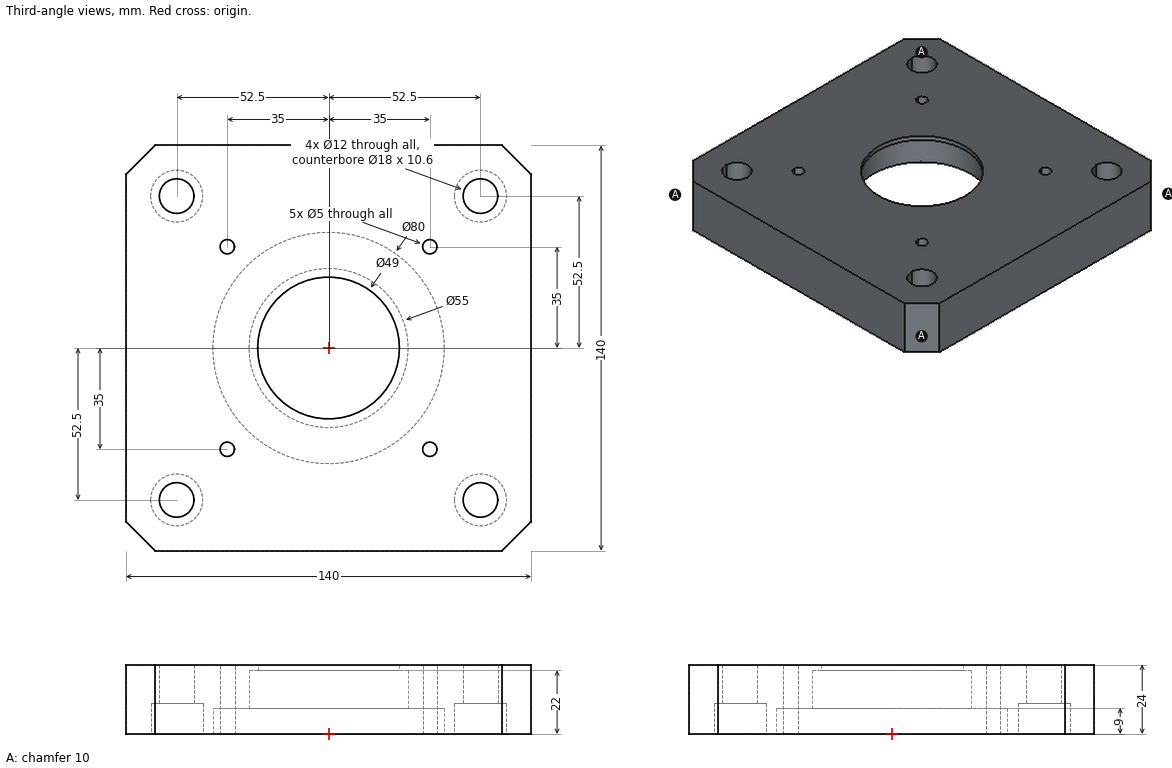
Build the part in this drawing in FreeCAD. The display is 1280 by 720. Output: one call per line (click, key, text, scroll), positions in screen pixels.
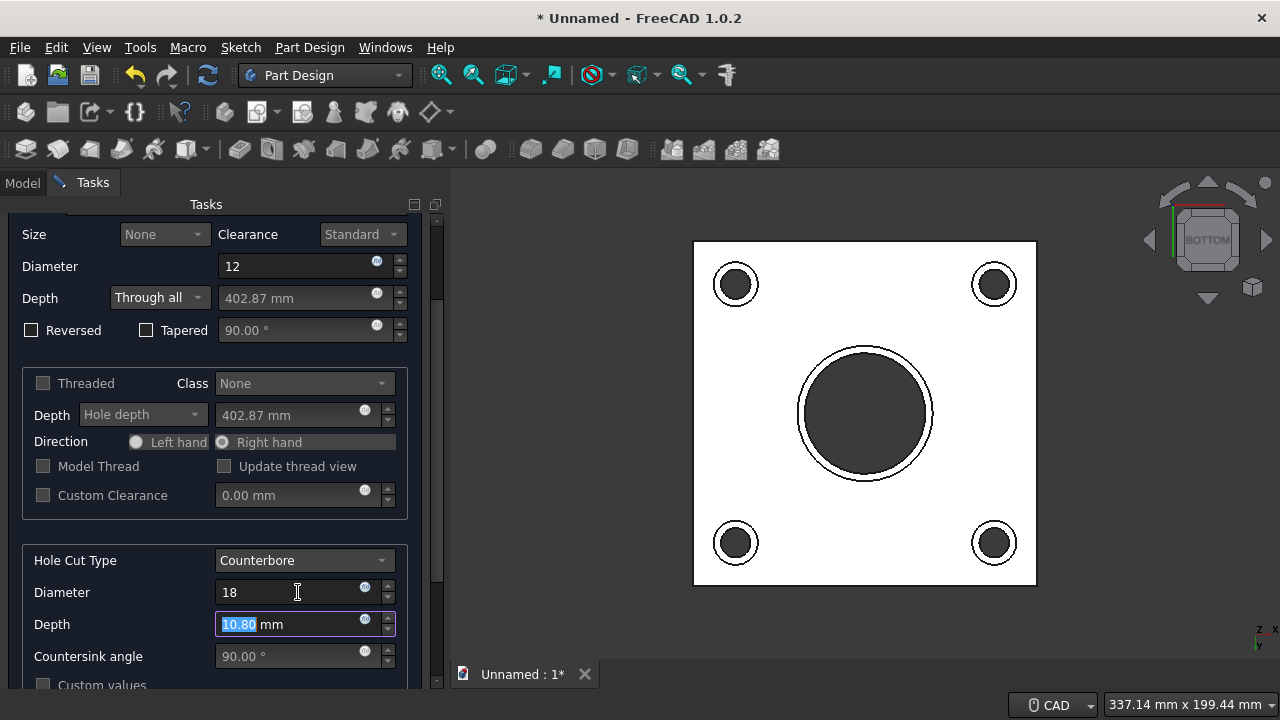
text(10.6)
key(Tab)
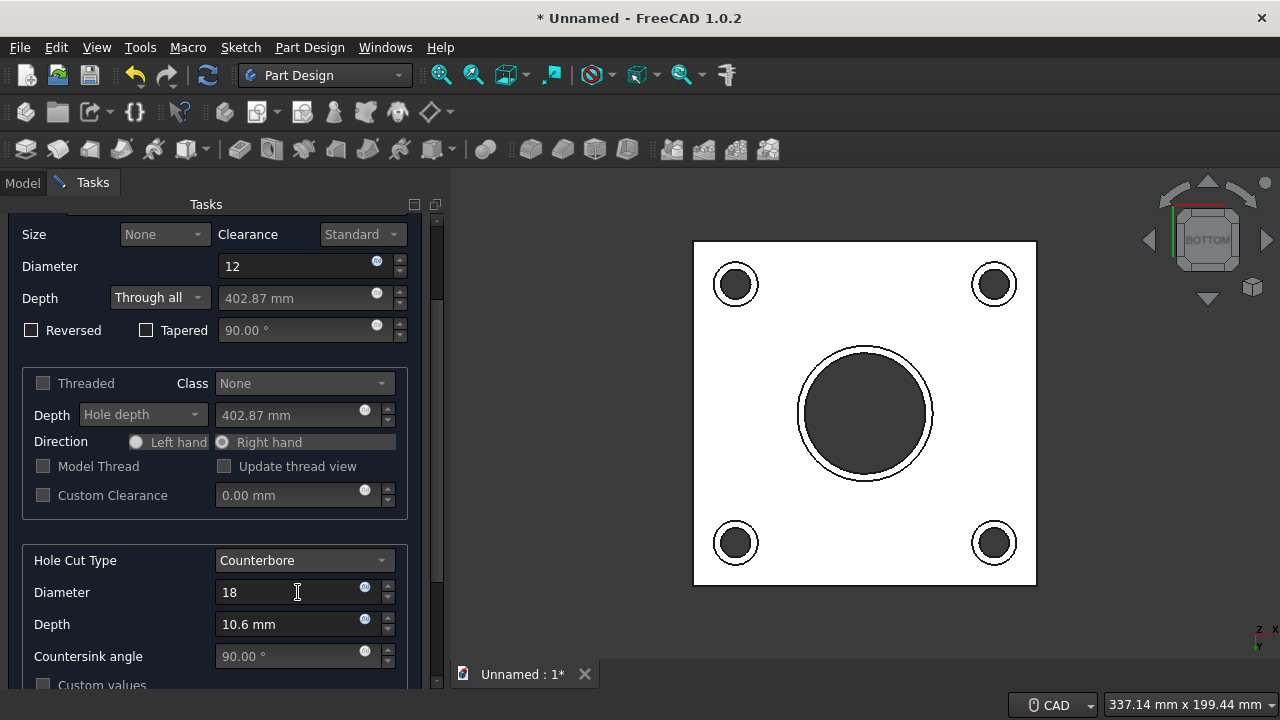
scroll(437, 451, up, 3)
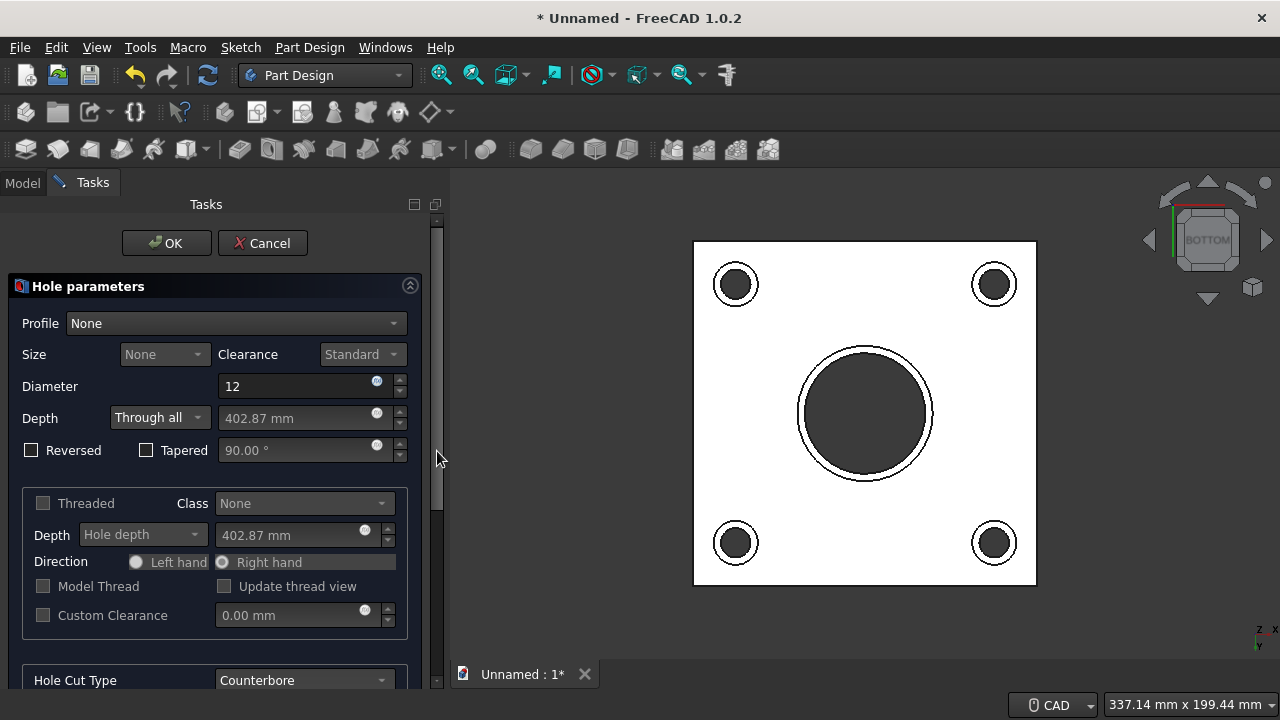
click(167, 243)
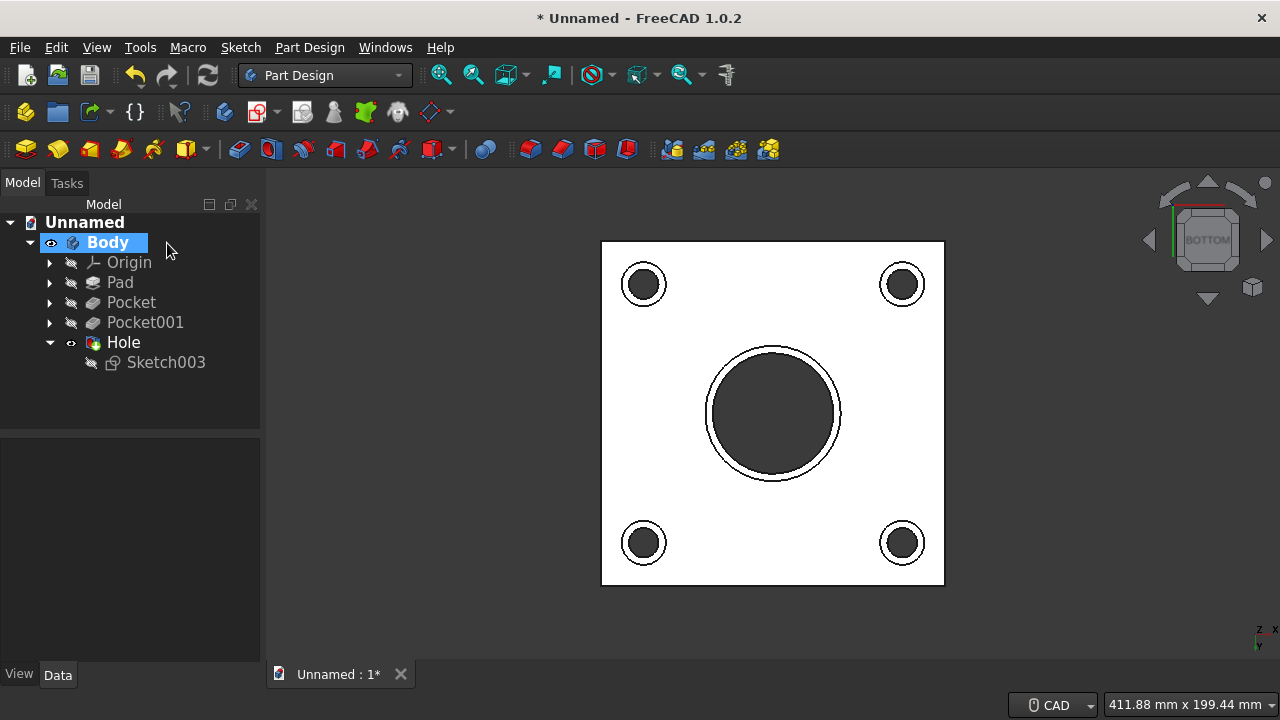
key(0)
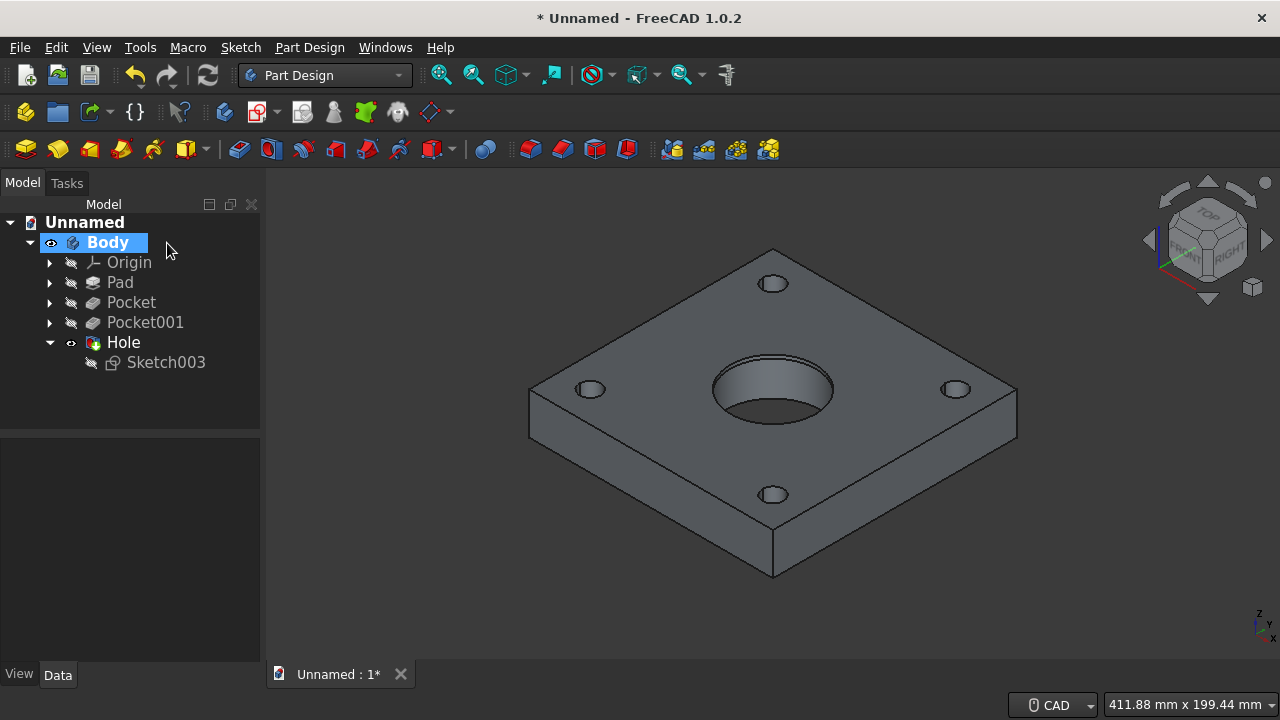
click(773, 553)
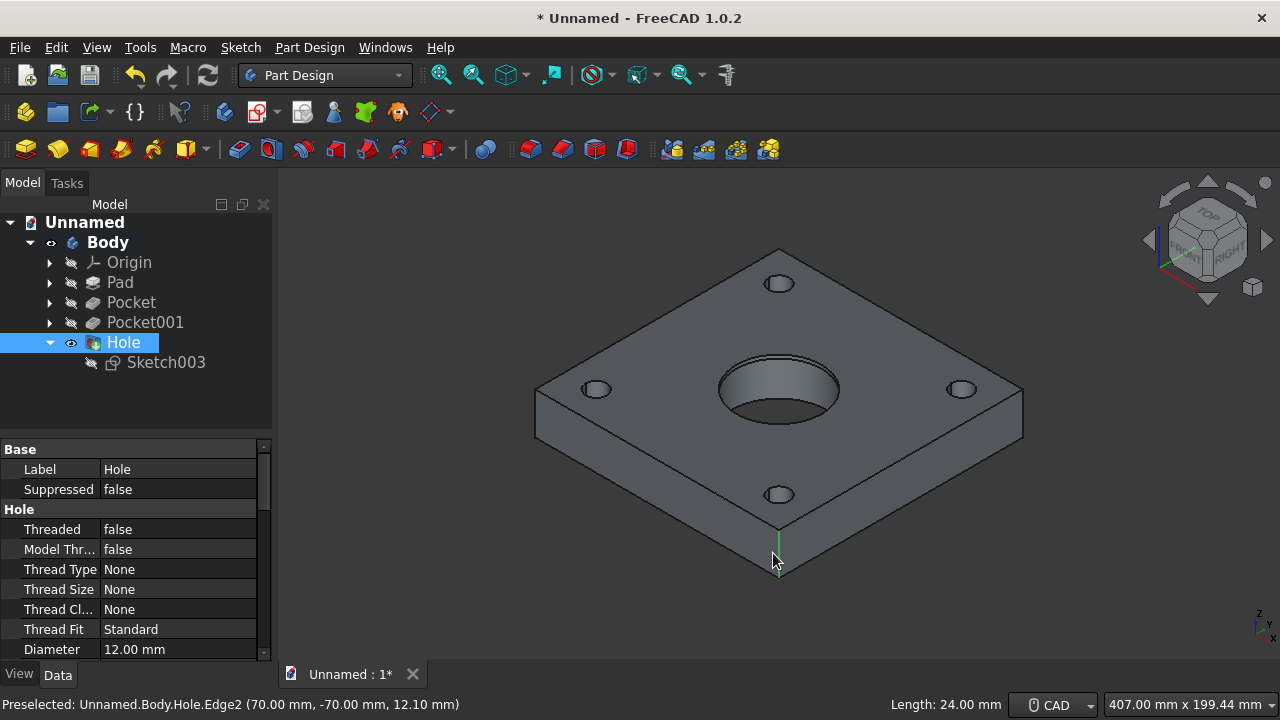
key(2)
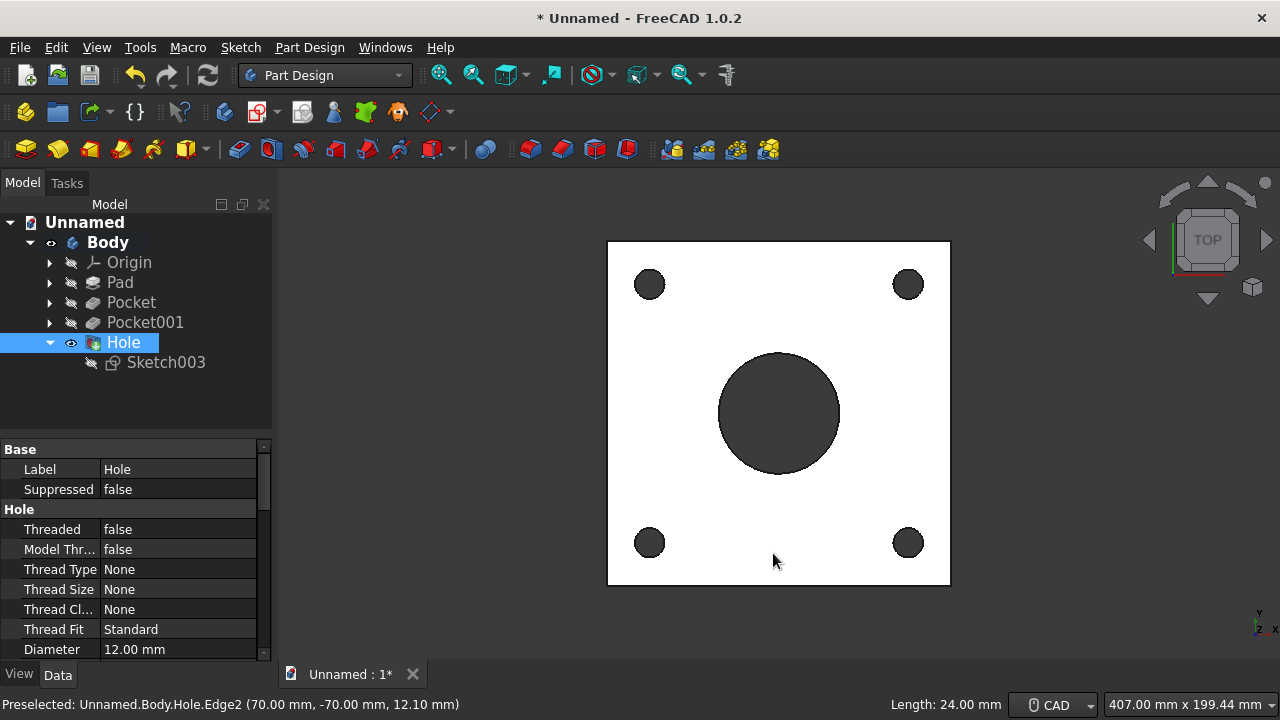
key(1)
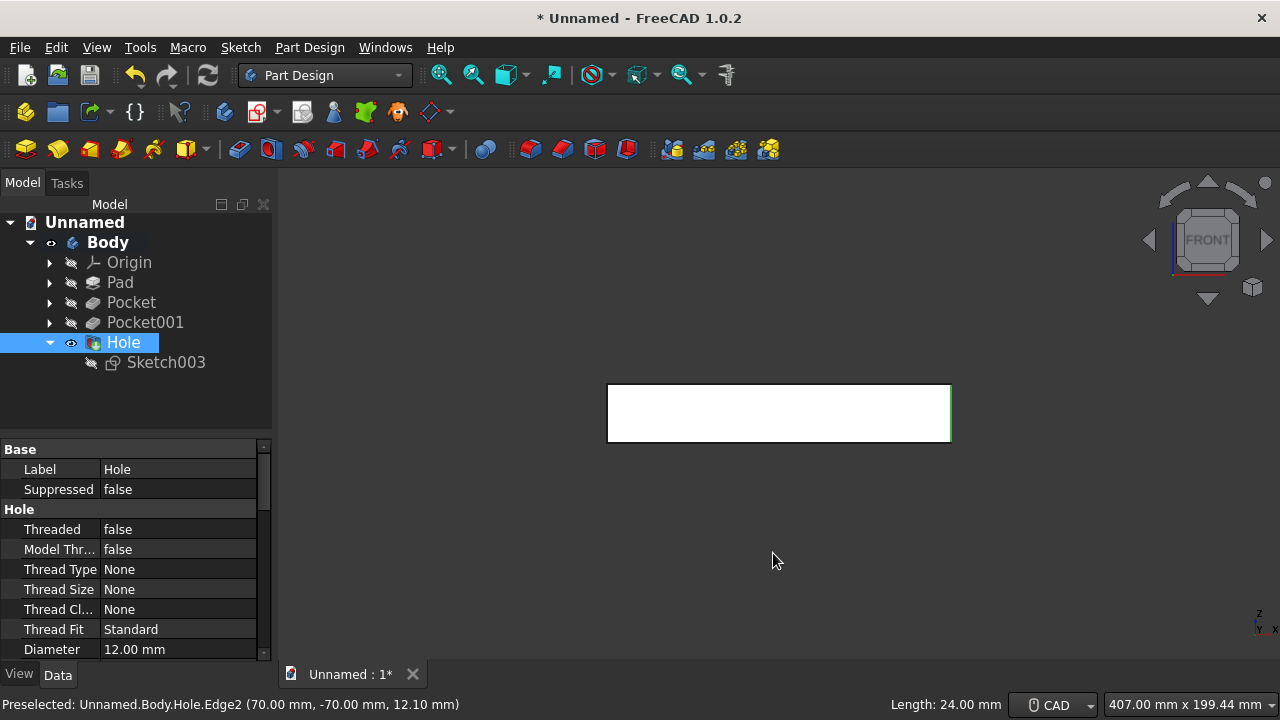
click(442, 76)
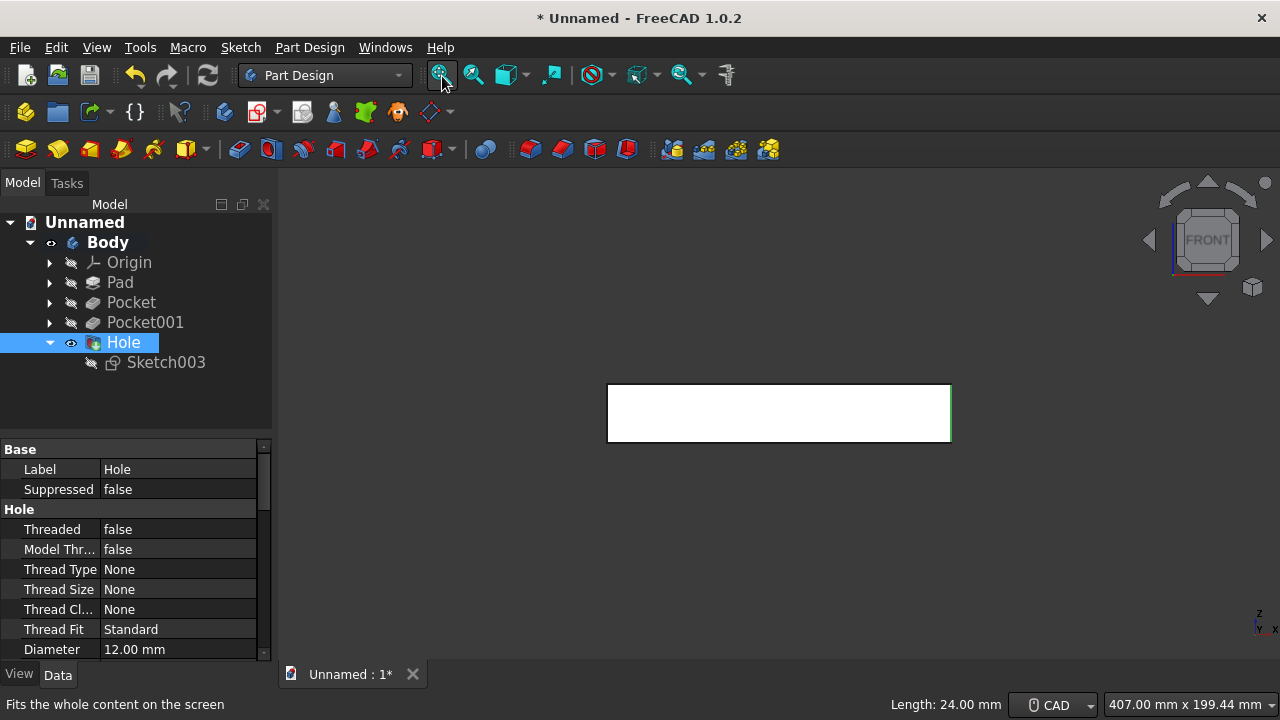
click(607, 413, ctrl)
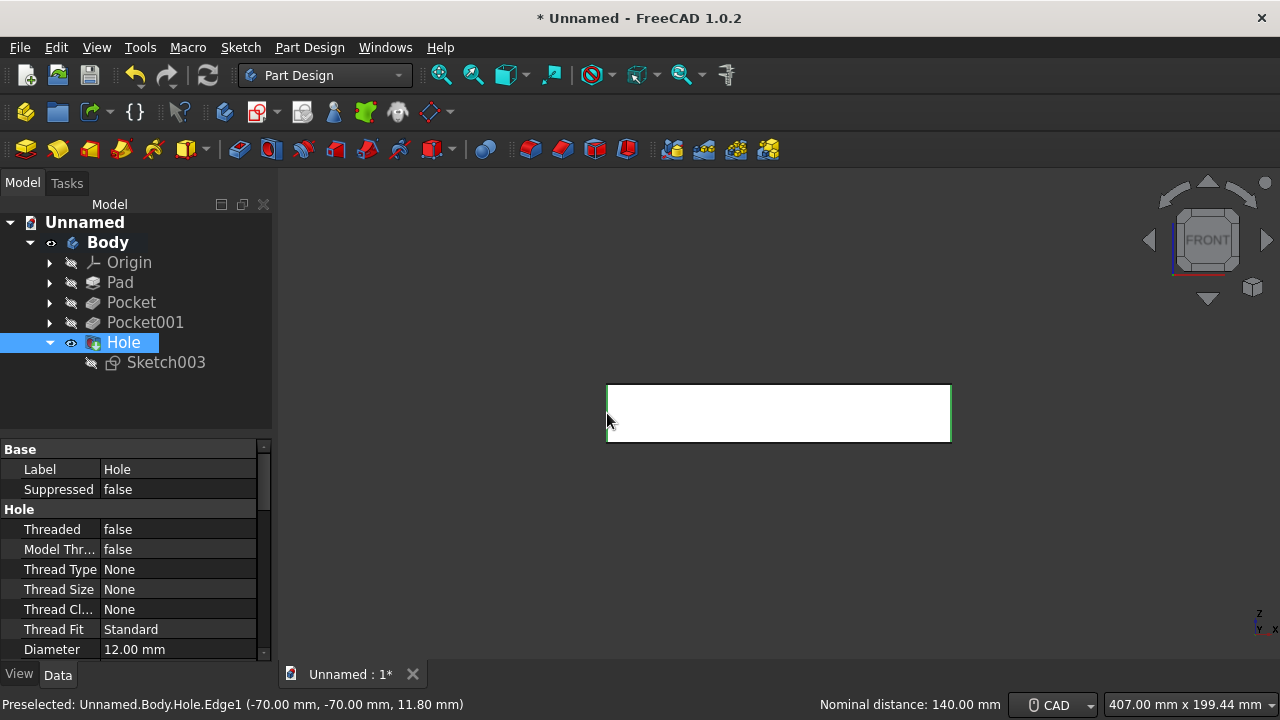
key(3)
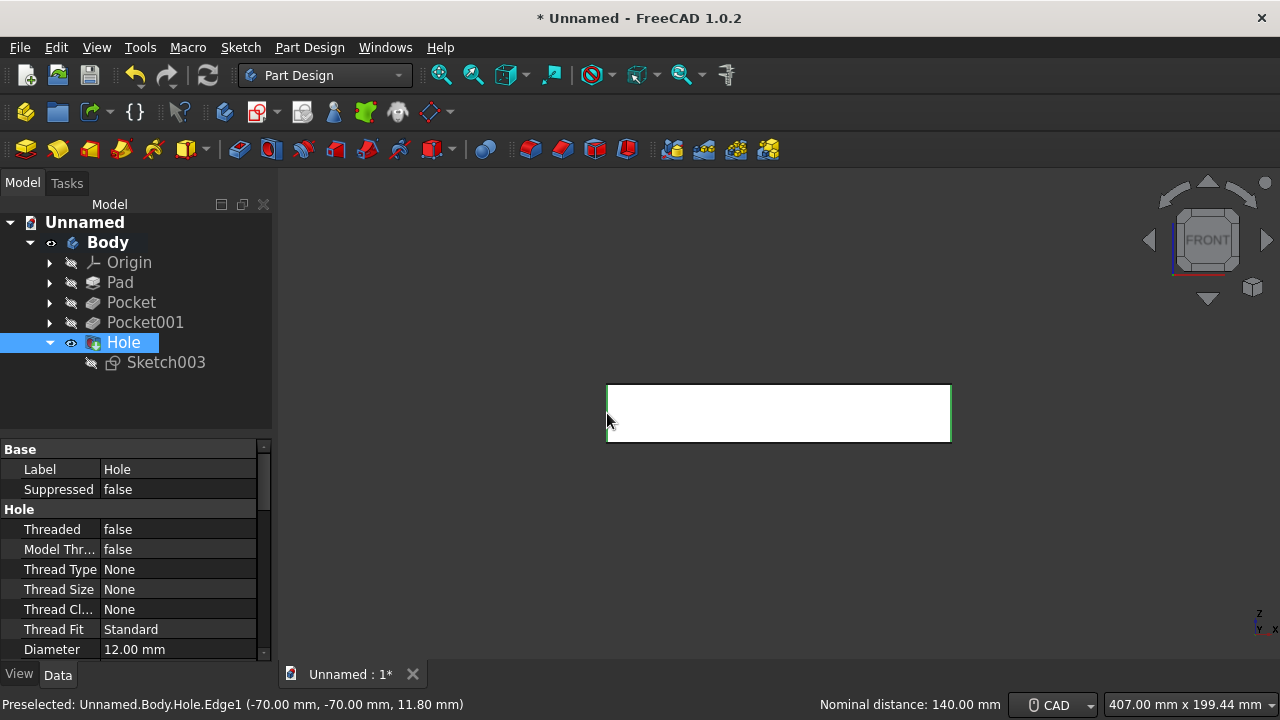
click(442, 76)